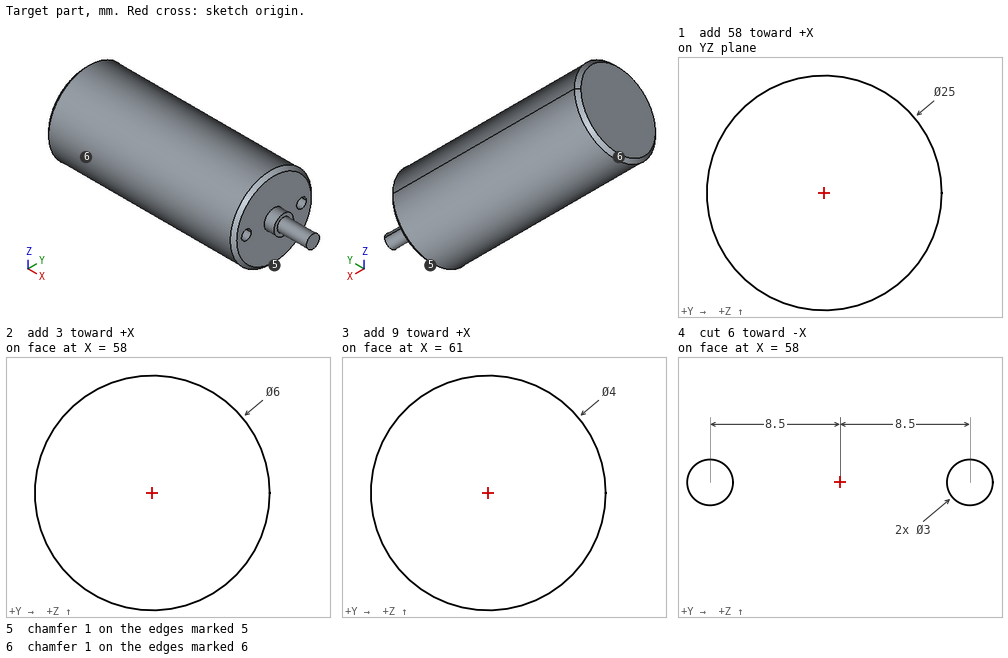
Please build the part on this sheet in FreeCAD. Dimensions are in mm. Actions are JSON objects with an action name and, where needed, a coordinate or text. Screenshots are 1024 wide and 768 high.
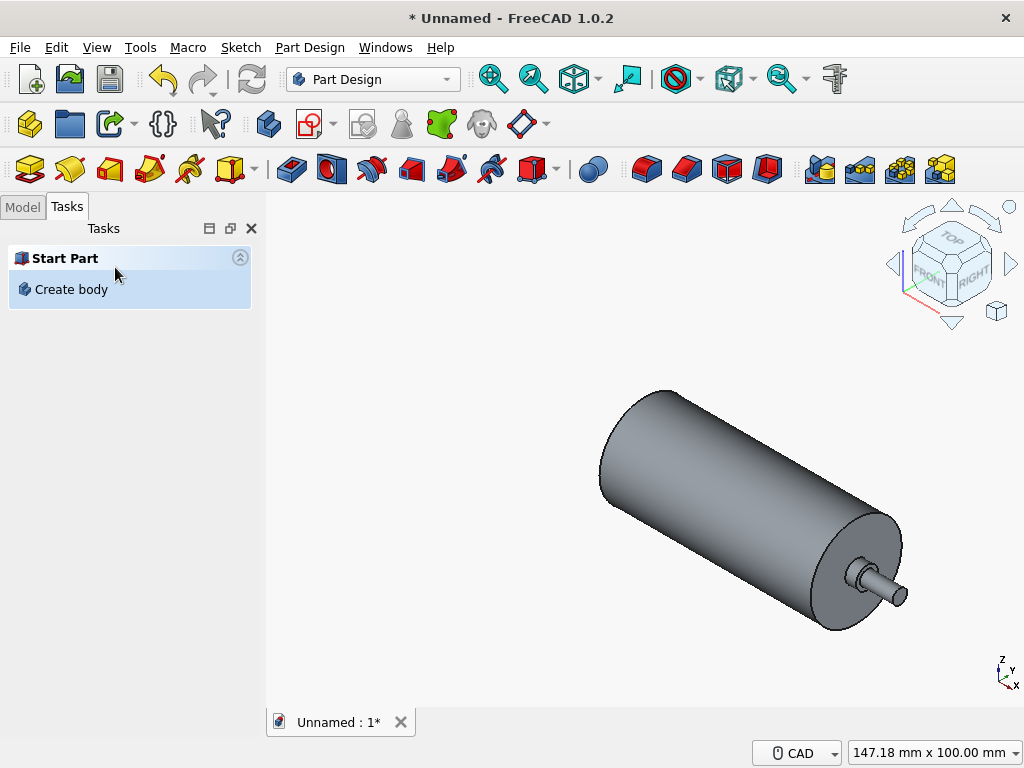
{"action": "left_click", "coordinate": [830, 570]}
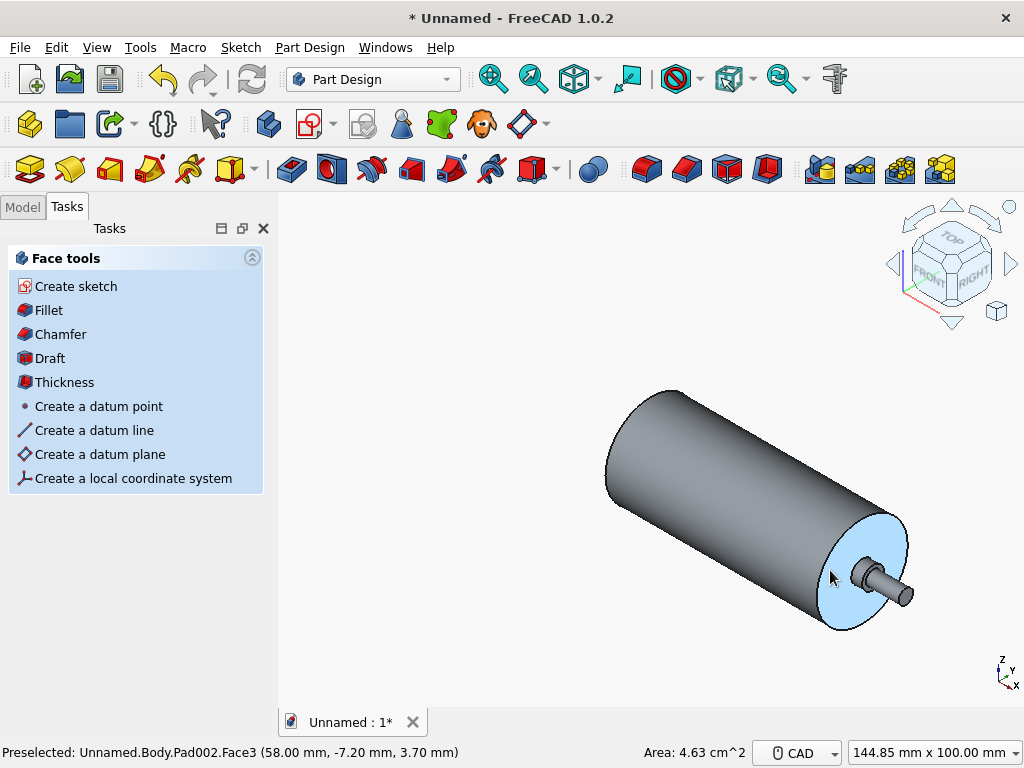
{"action": "left_click", "coordinate": [310, 124]}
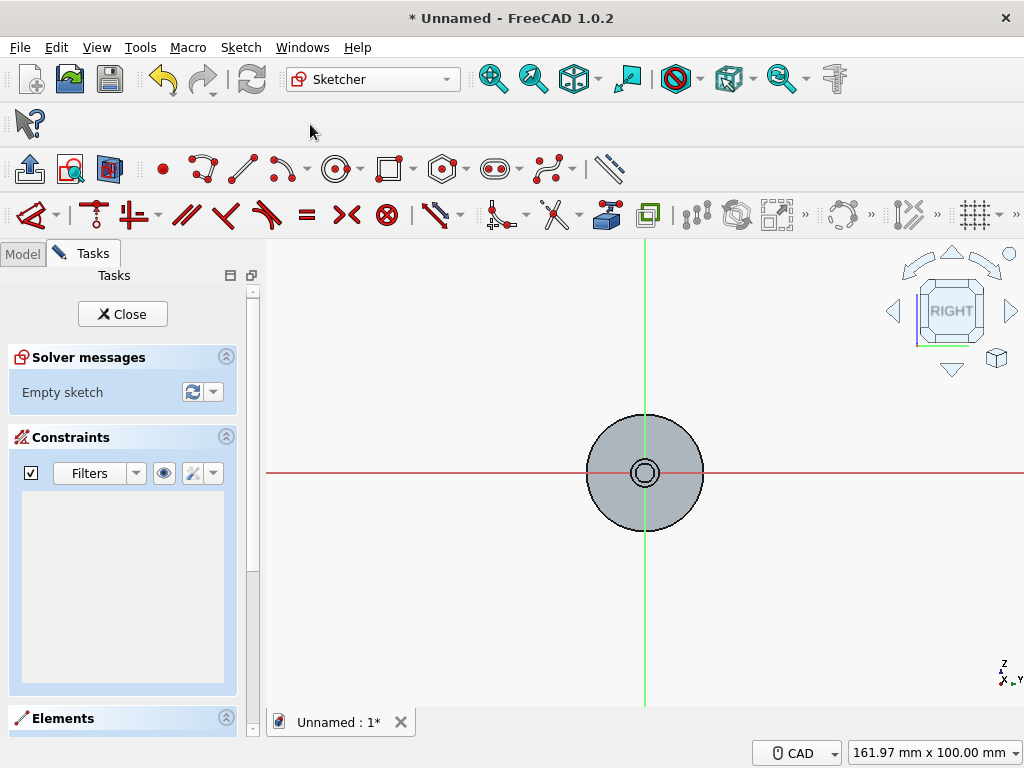
{"action": "left_click", "coordinate": [110, 170]}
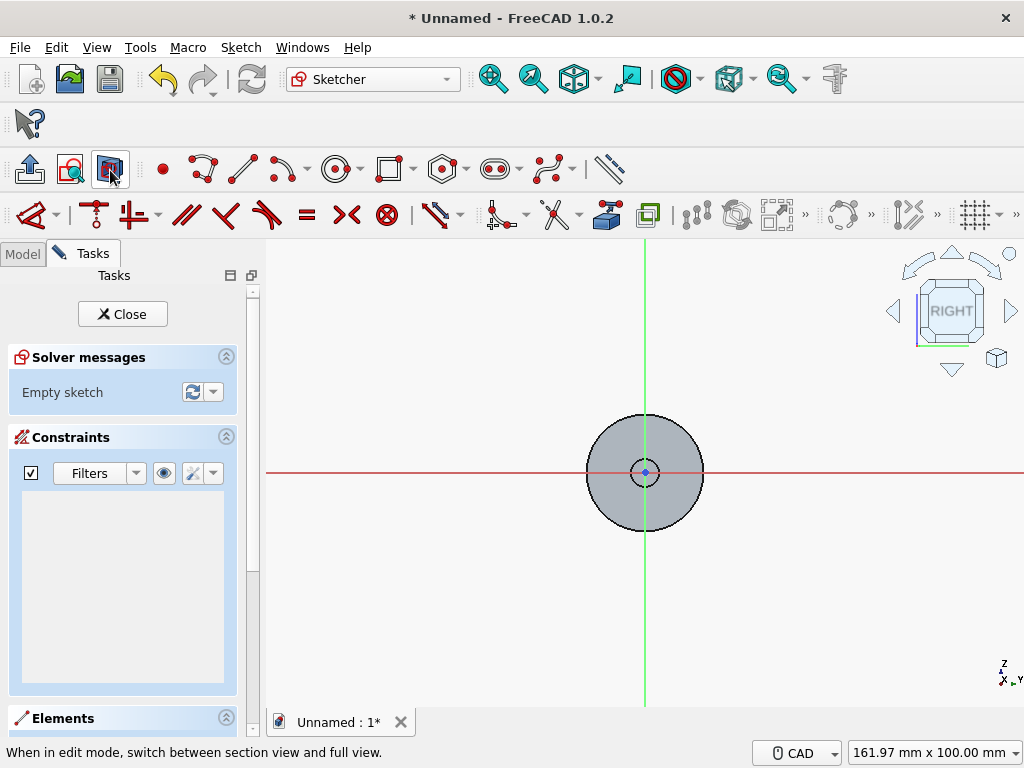
{"action": "scroll", "coordinate": [667, 473], "scroll_direction": "up", "scroll_amount": 7}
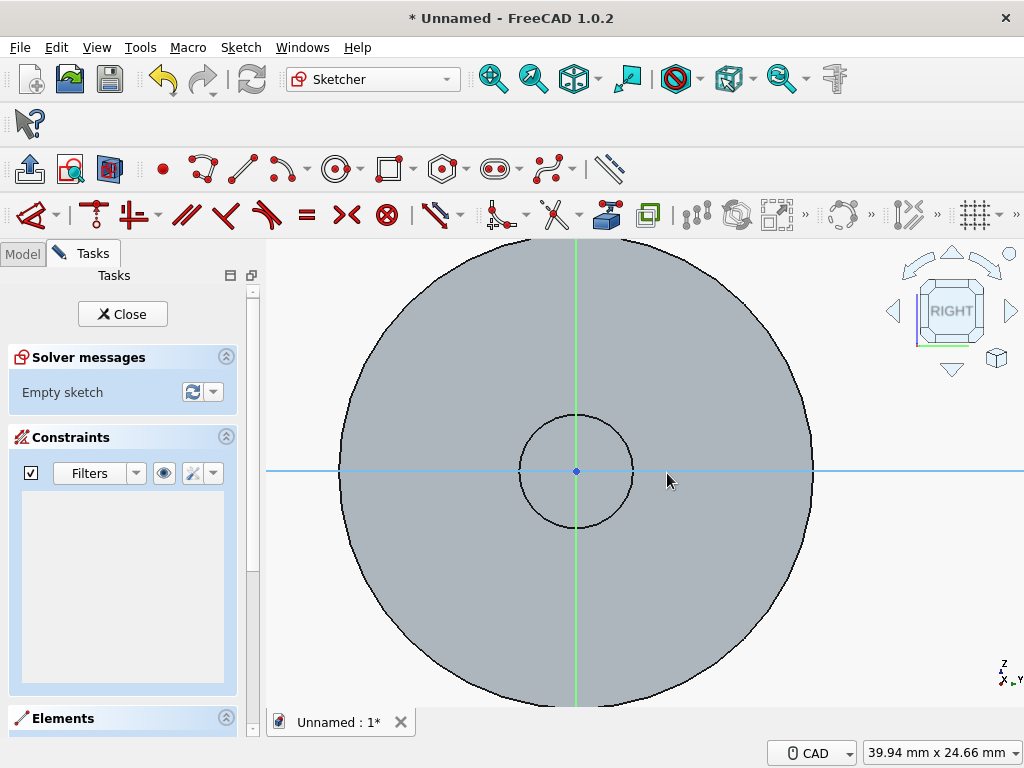
{"action": "left_click", "coordinate": [336, 170]}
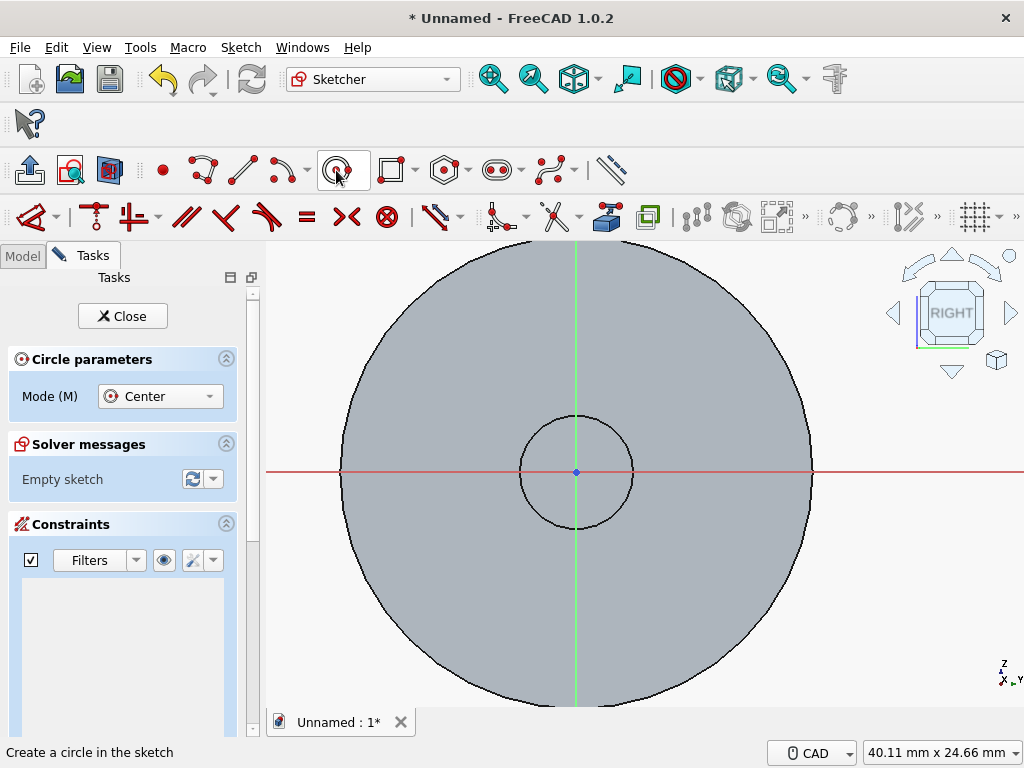
{"action": "left_click", "coordinate": [737, 472]}
{"action": "left_click", "coordinate": [757, 452]}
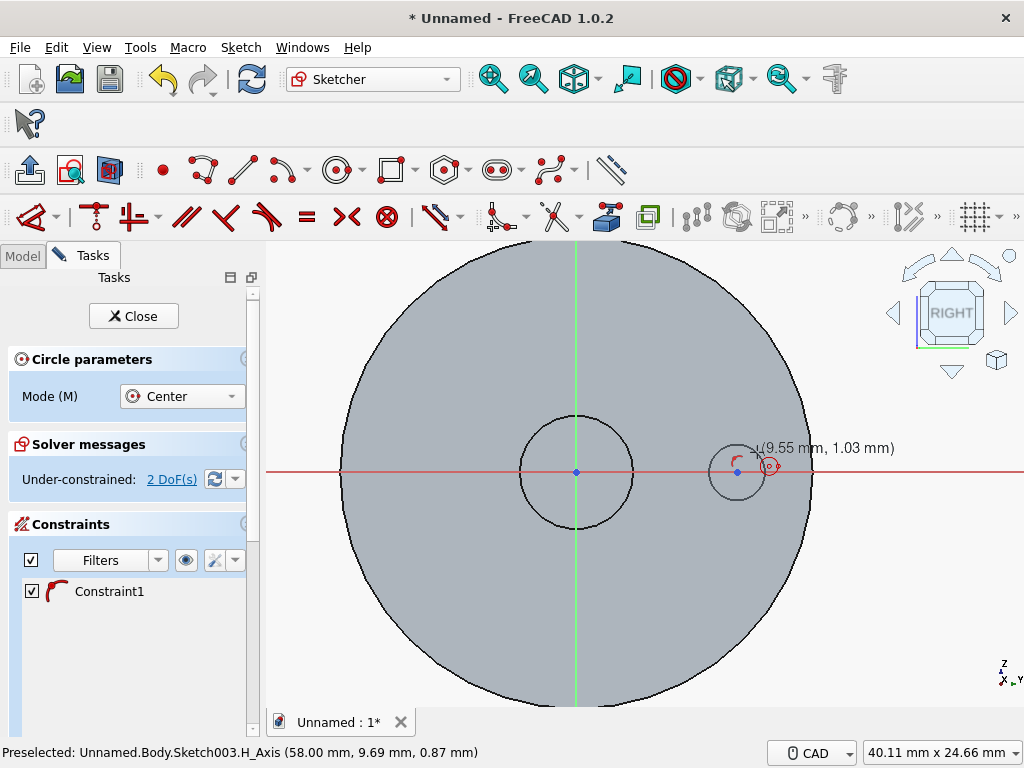
{"action": "left_click", "coordinate": [416, 472]}
{"action": "left_click", "coordinate": [436, 452]}
{"action": "key", "text": "Escape"}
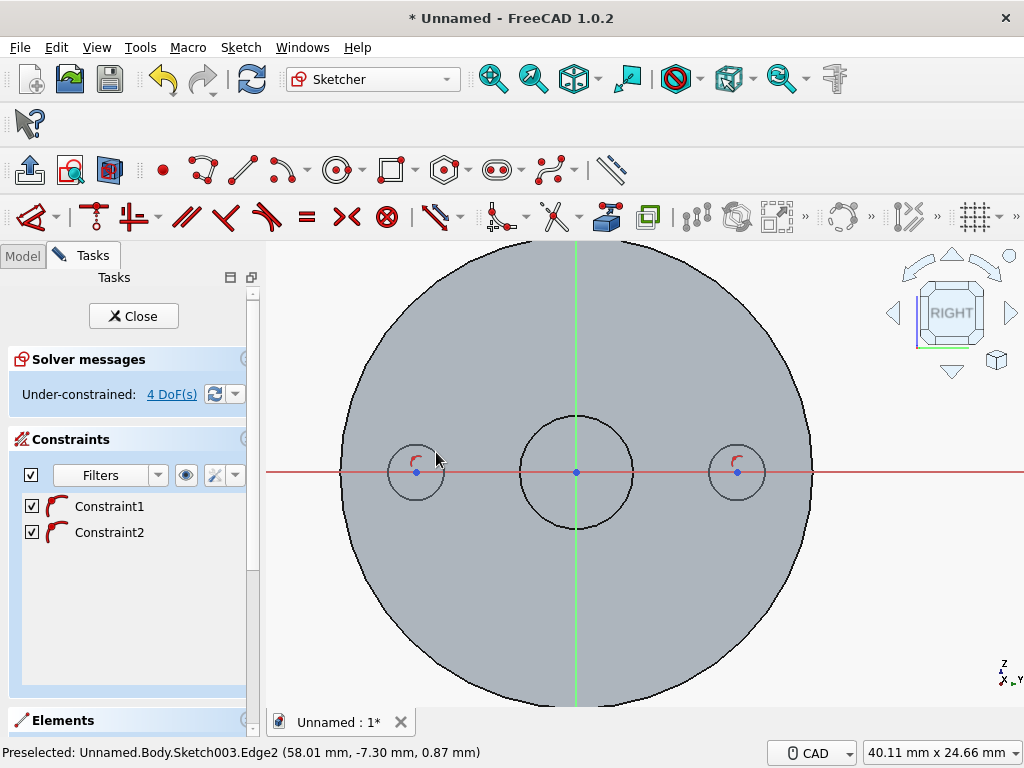
{"action": "left_click", "coordinate": [757, 453]}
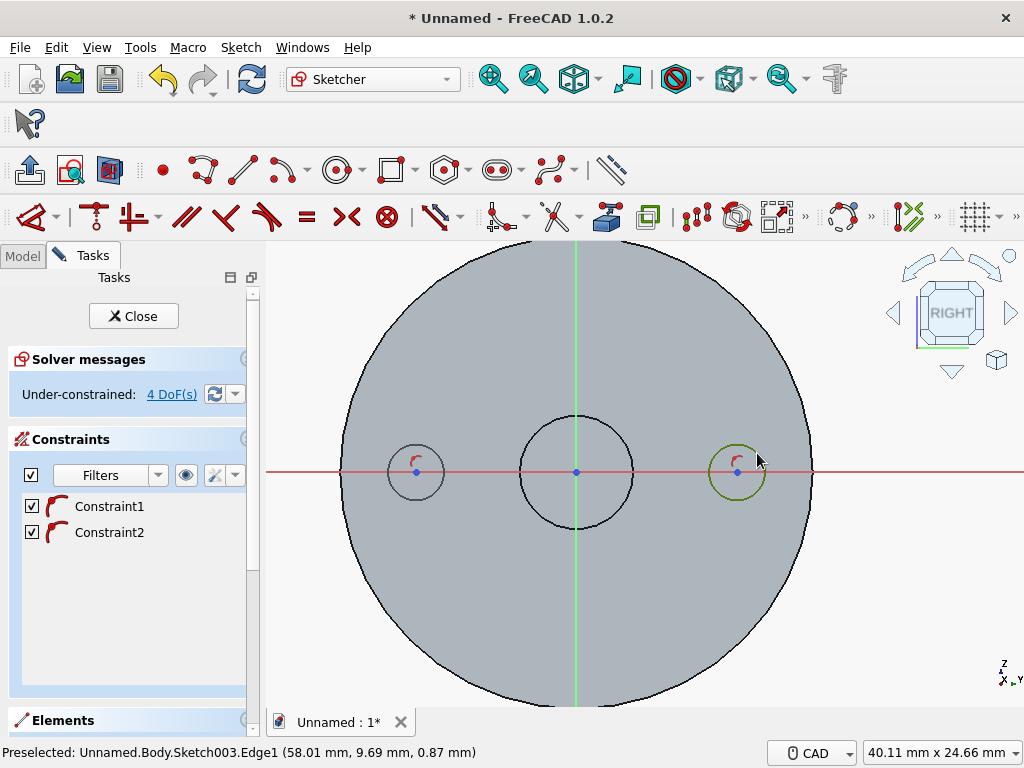
{"action": "left_click", "coordinate": [436, 453]}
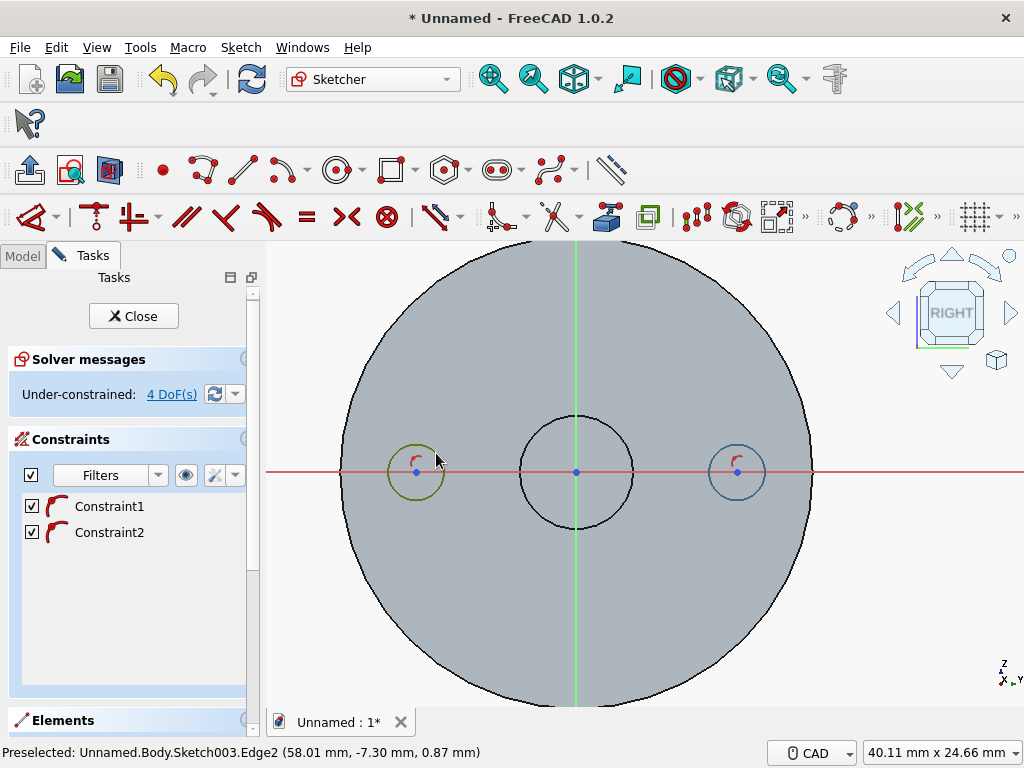
{"action": "key", "text": "e"}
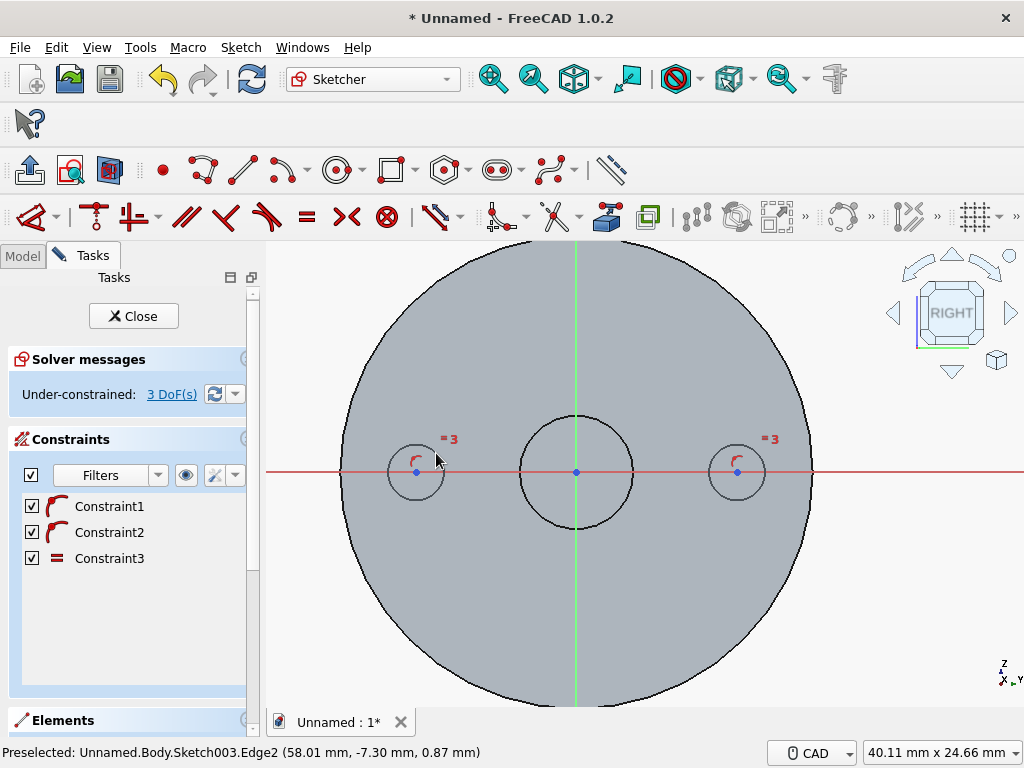
{"action": "key", "text": "d"}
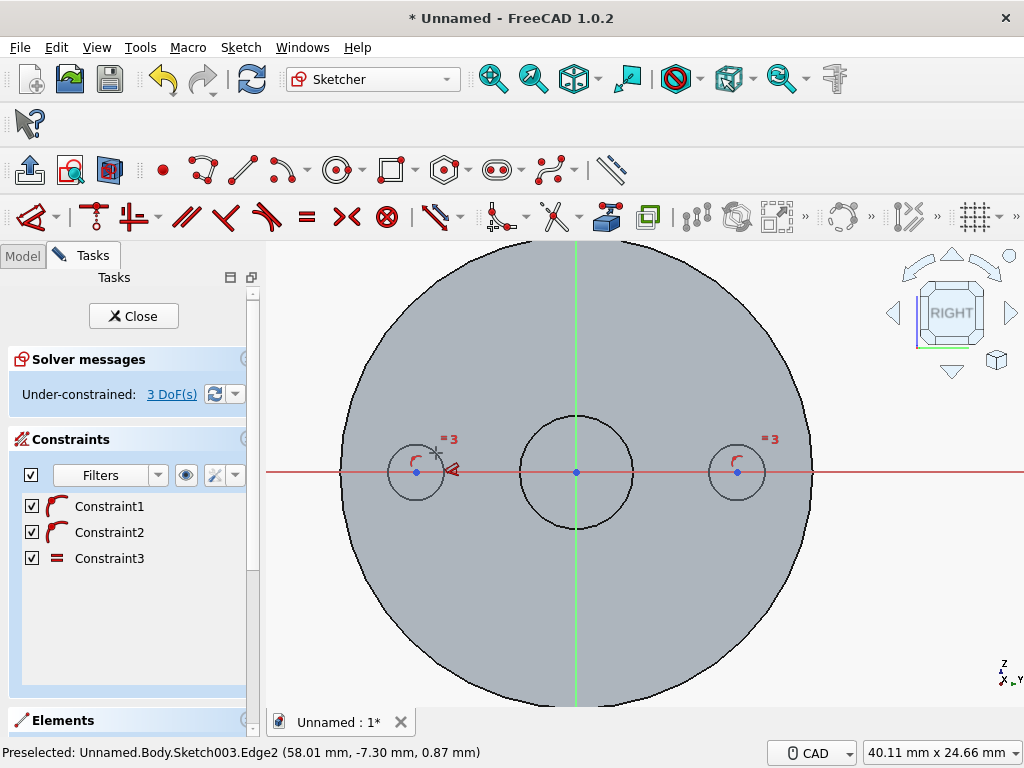
{"action": "left_click", "coordinate": [757, 453]}
{"action": "left_click", "coordinate": [780, 431]}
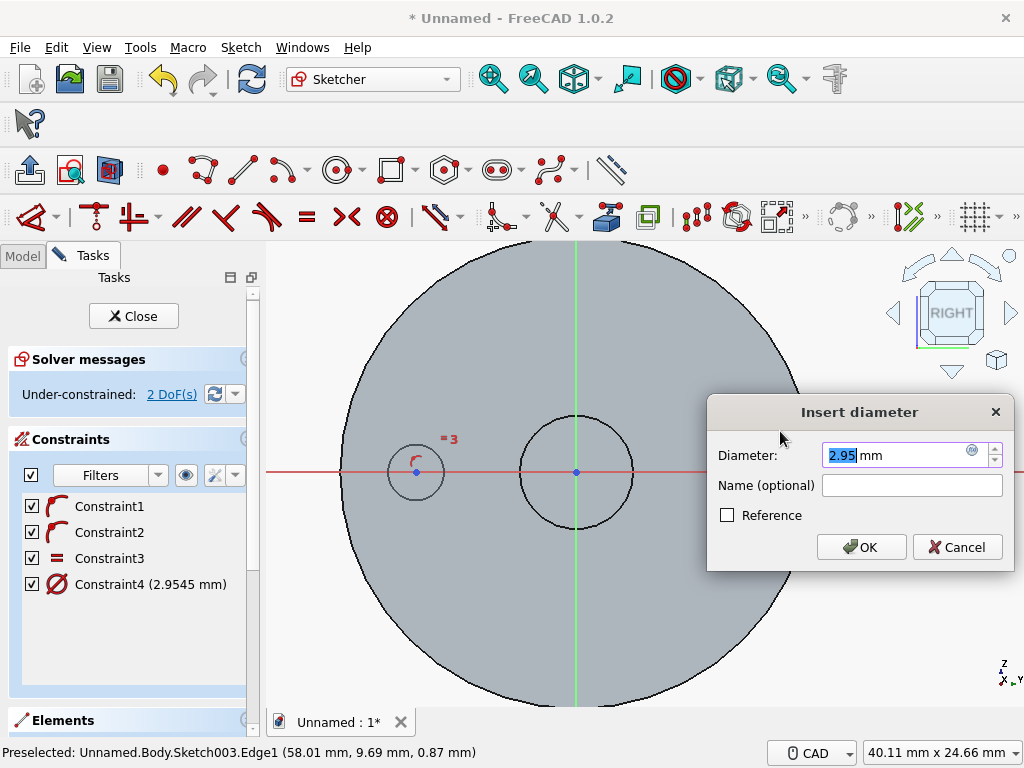
{"action": "type", "text": "3"}
{"action": "key", "text": "Return"}